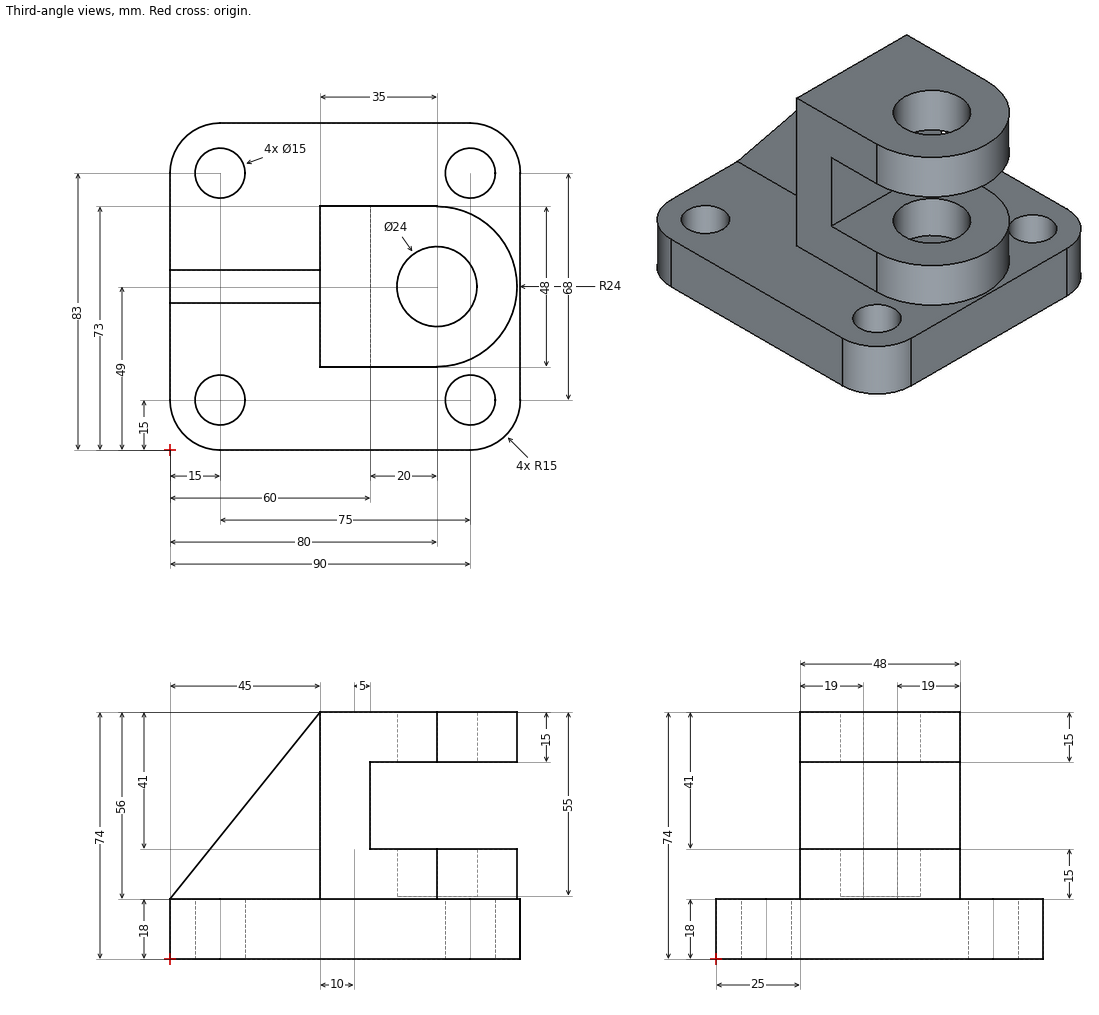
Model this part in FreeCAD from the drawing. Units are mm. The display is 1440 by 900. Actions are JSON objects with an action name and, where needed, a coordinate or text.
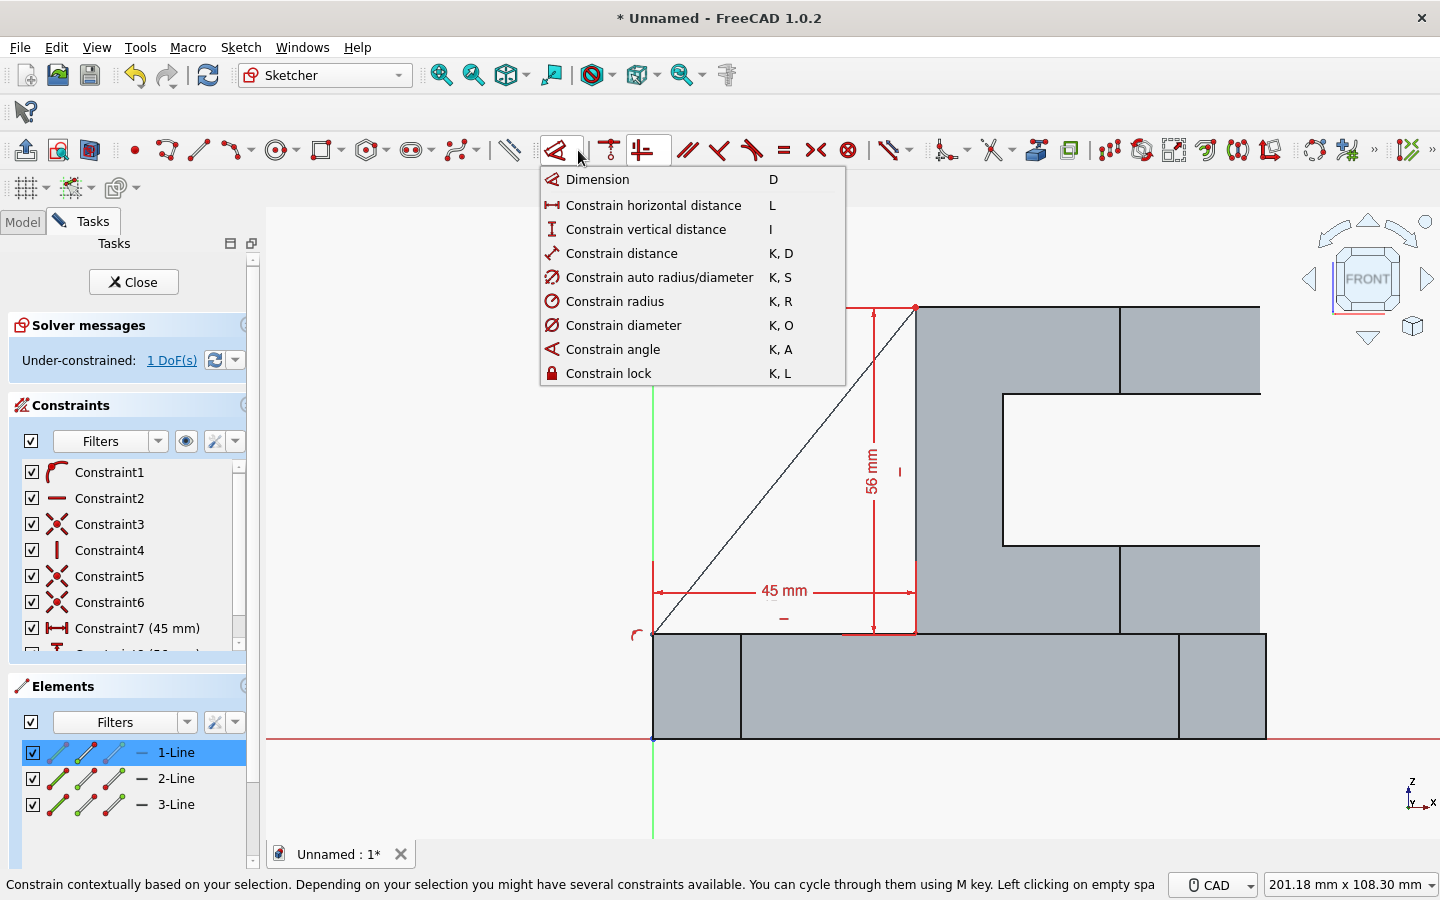
{"action": "left_click", "coordinate": [693, 229]}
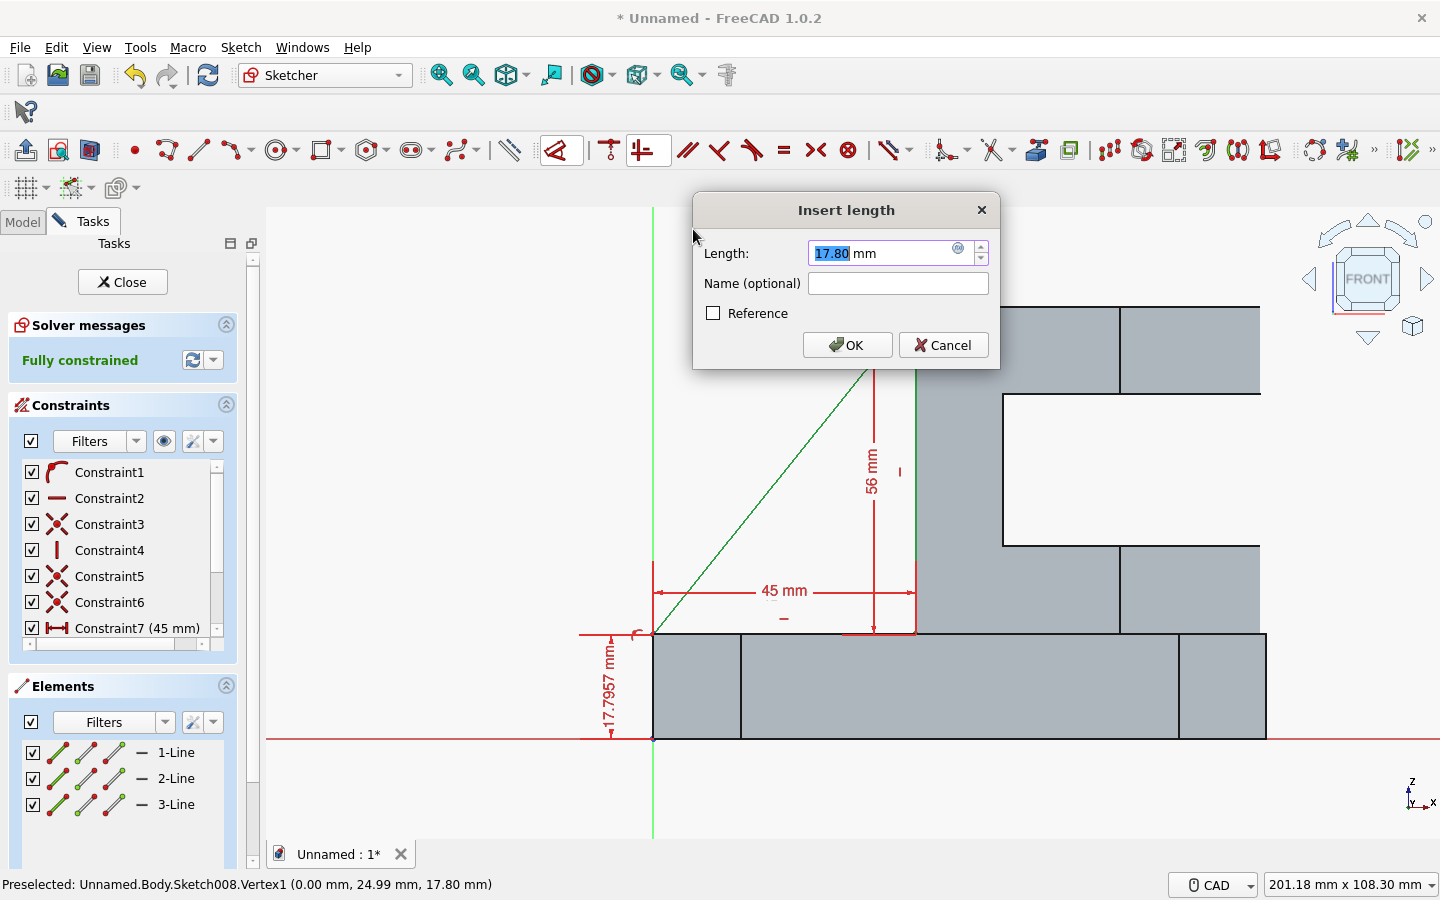
{"action": "type", "text": "18"}
{"action": "key", "text": "Return"}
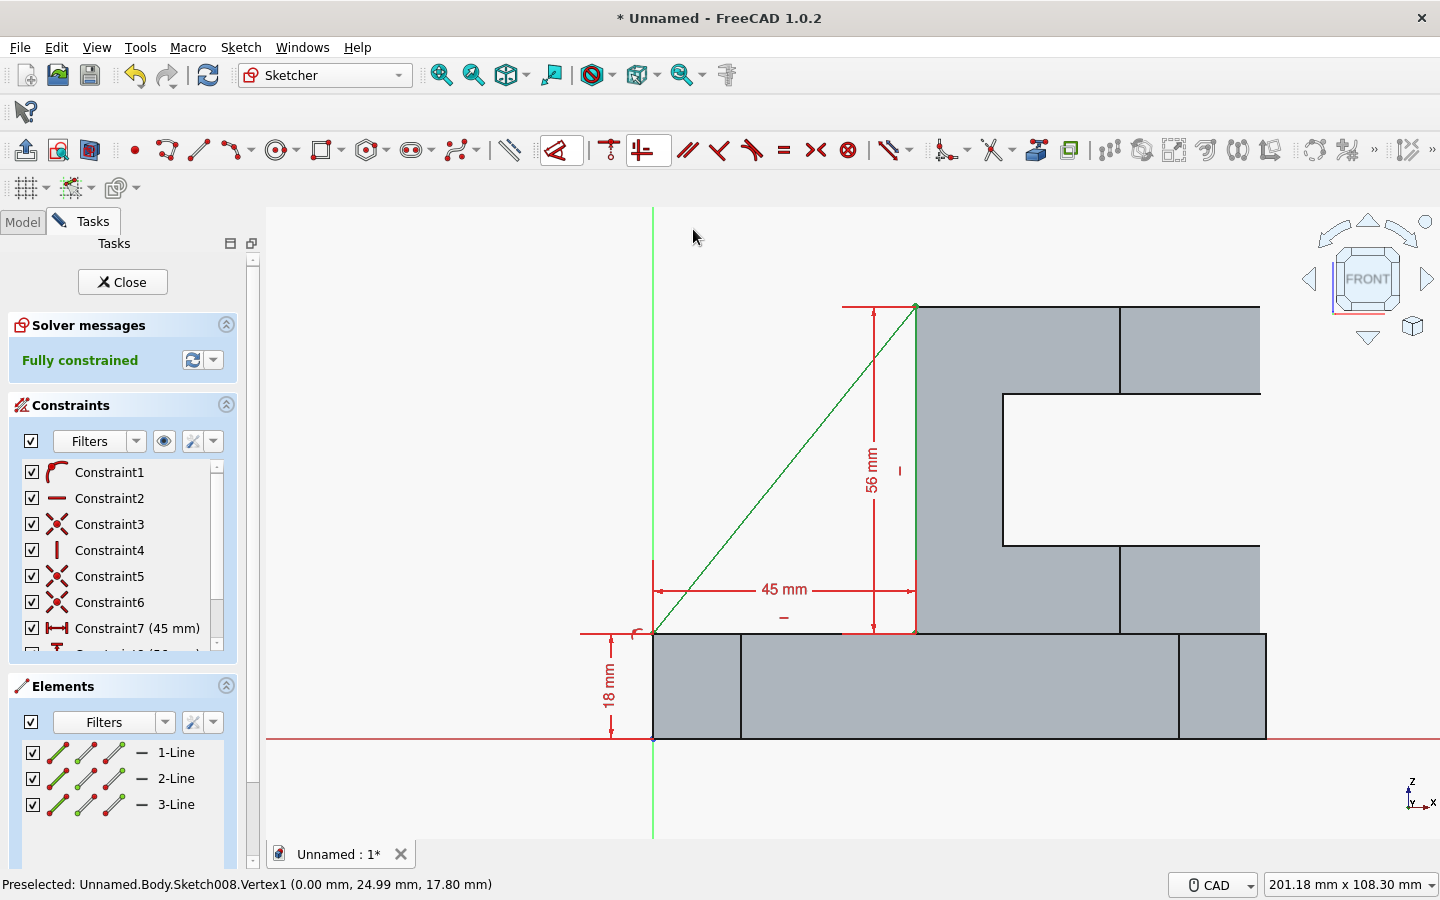
{"action": "left_click", "coordinate": [123, 282]}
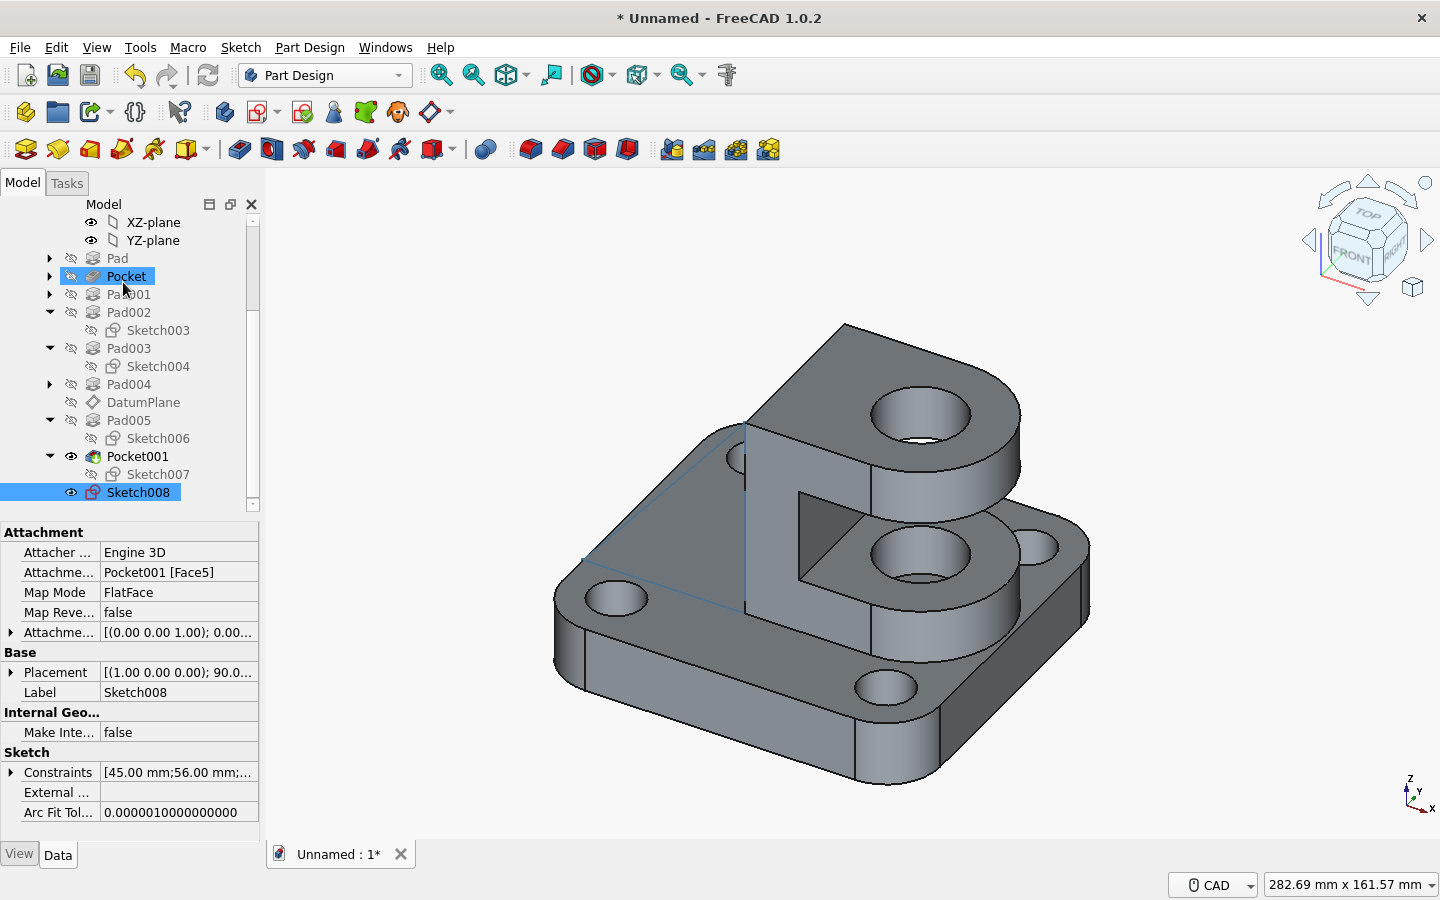
{"action": "left_click", "coordinate": [26, 150]}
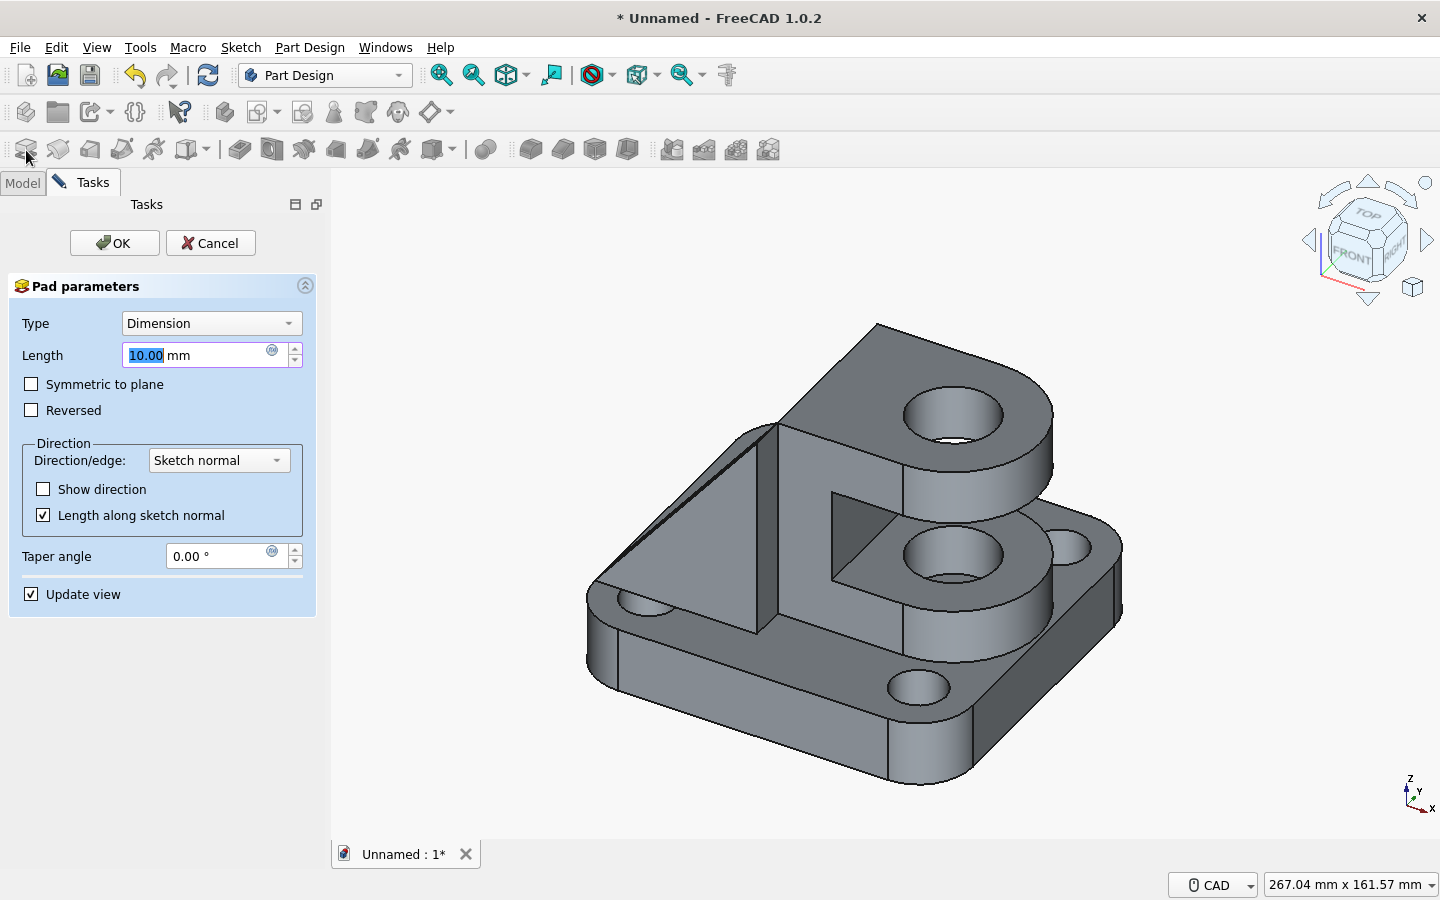
{"action": "type", "text": "48"}
{"action": "key", "text": "Tab"}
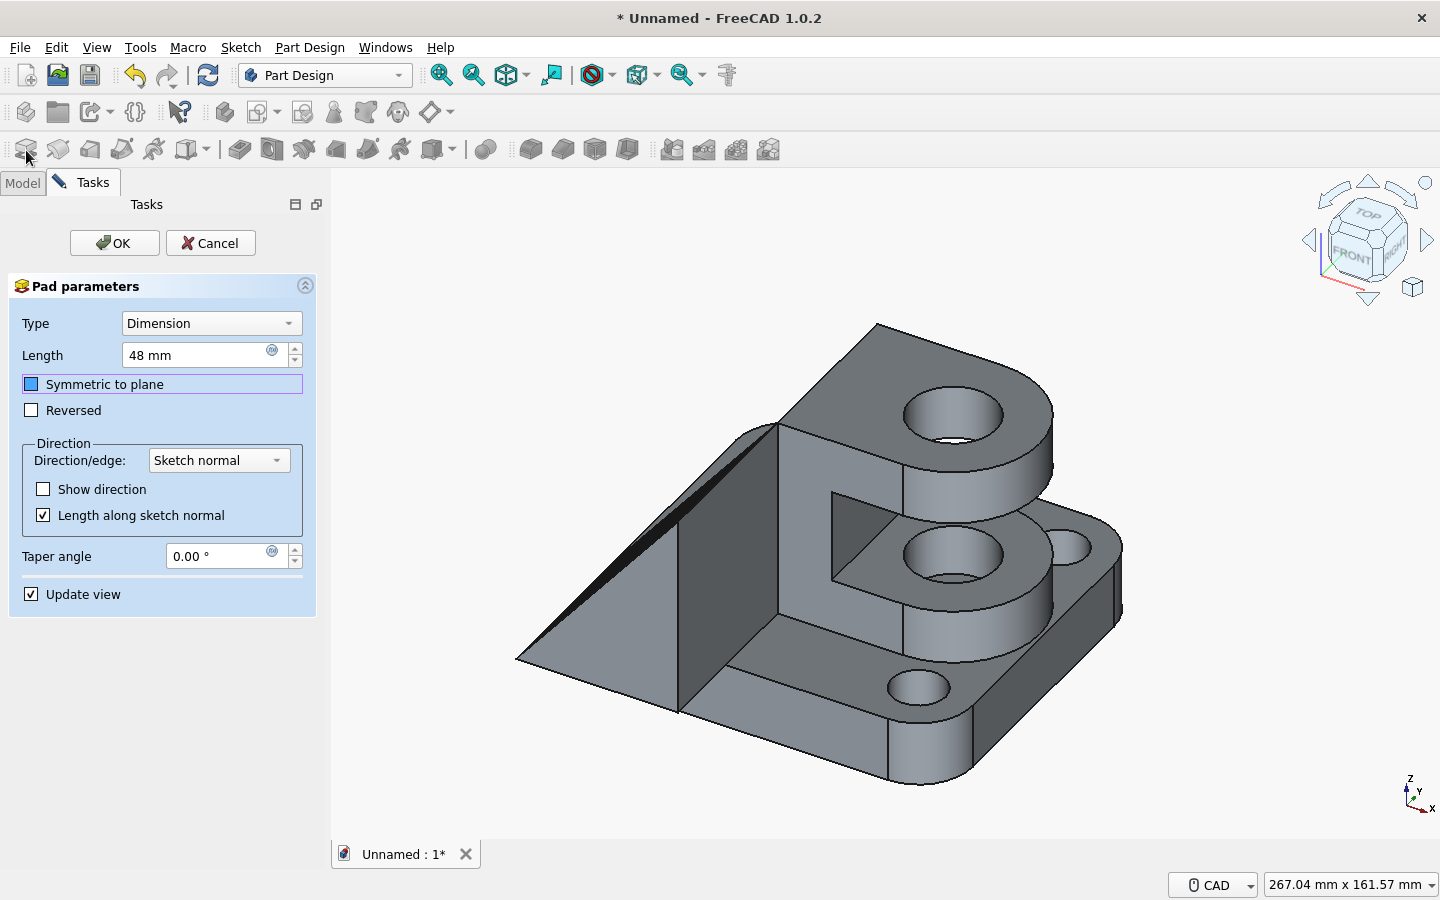
{"action": "left_click", "coordinate": [30, 410]}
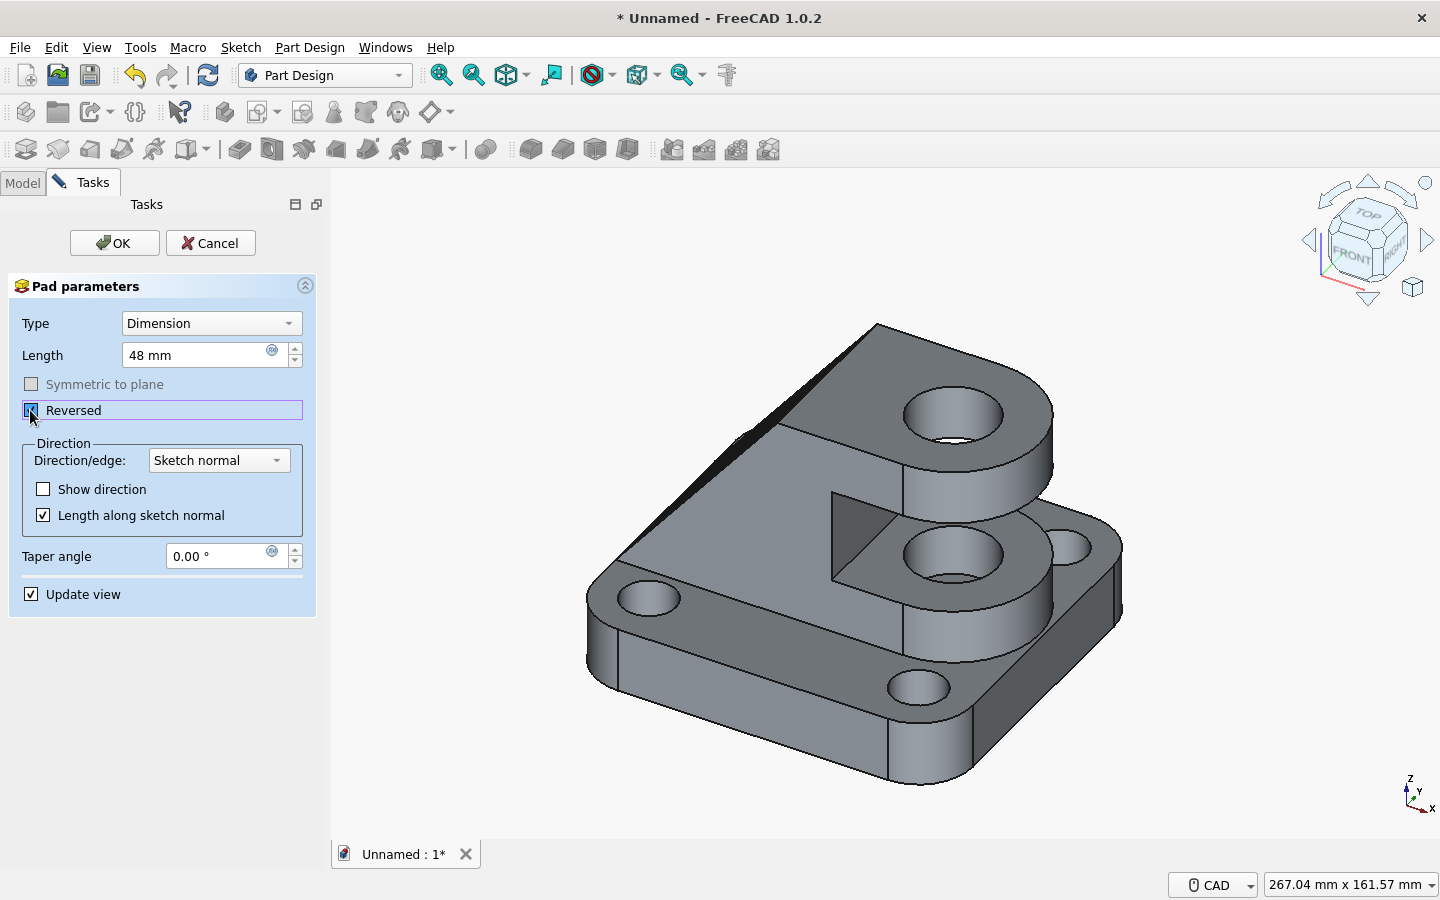
{"action": "left_click", "coordinate": [115, 243]}